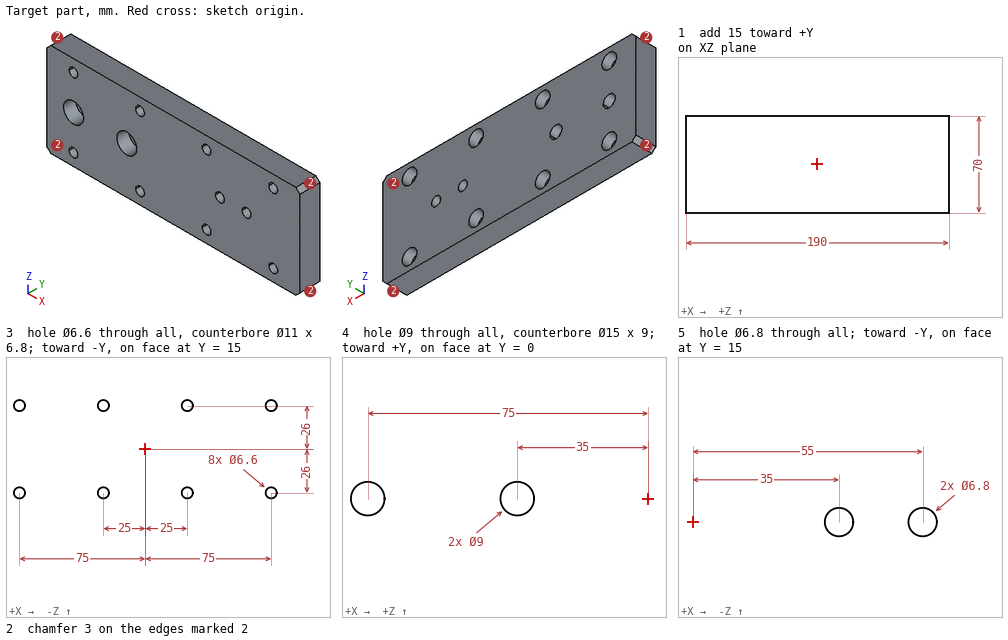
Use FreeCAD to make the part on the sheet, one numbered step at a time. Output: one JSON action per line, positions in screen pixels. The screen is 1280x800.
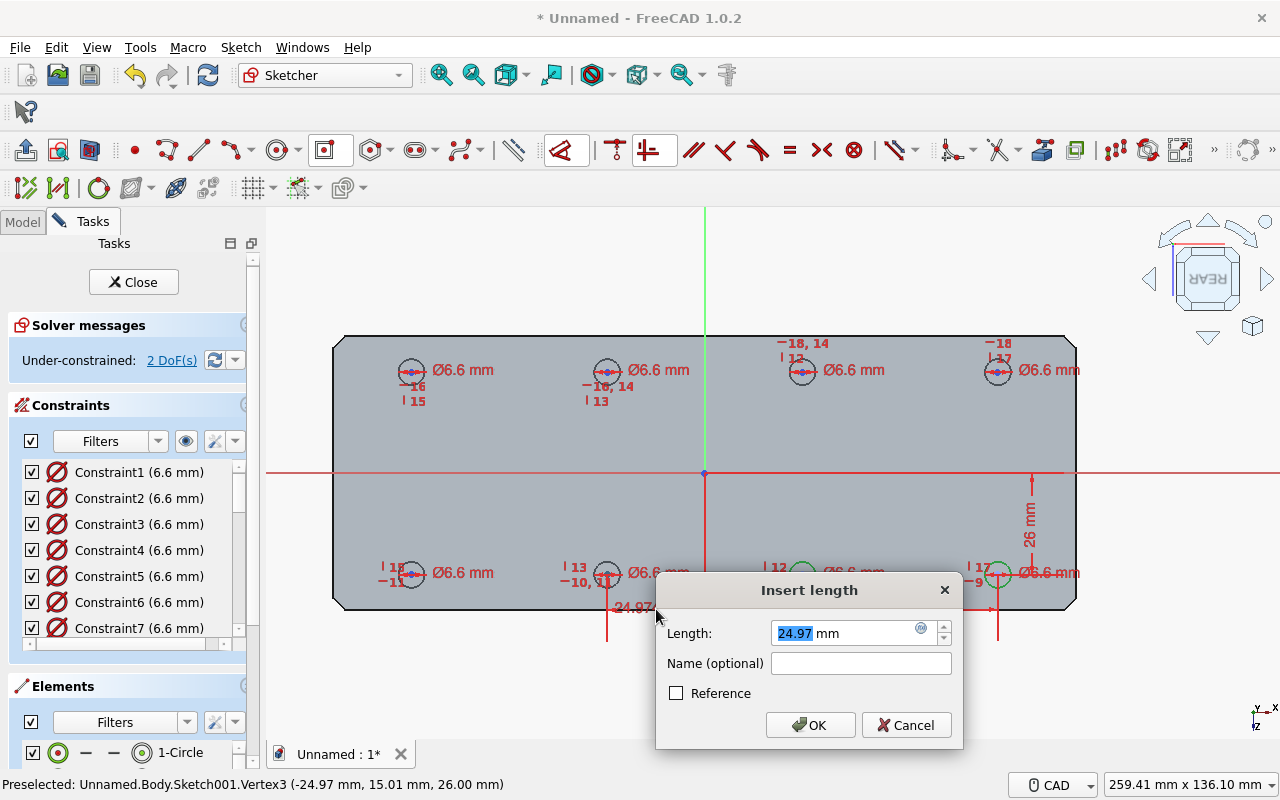
{"action": "type", "text": "25"}
{"action": "key", "text": "Return"}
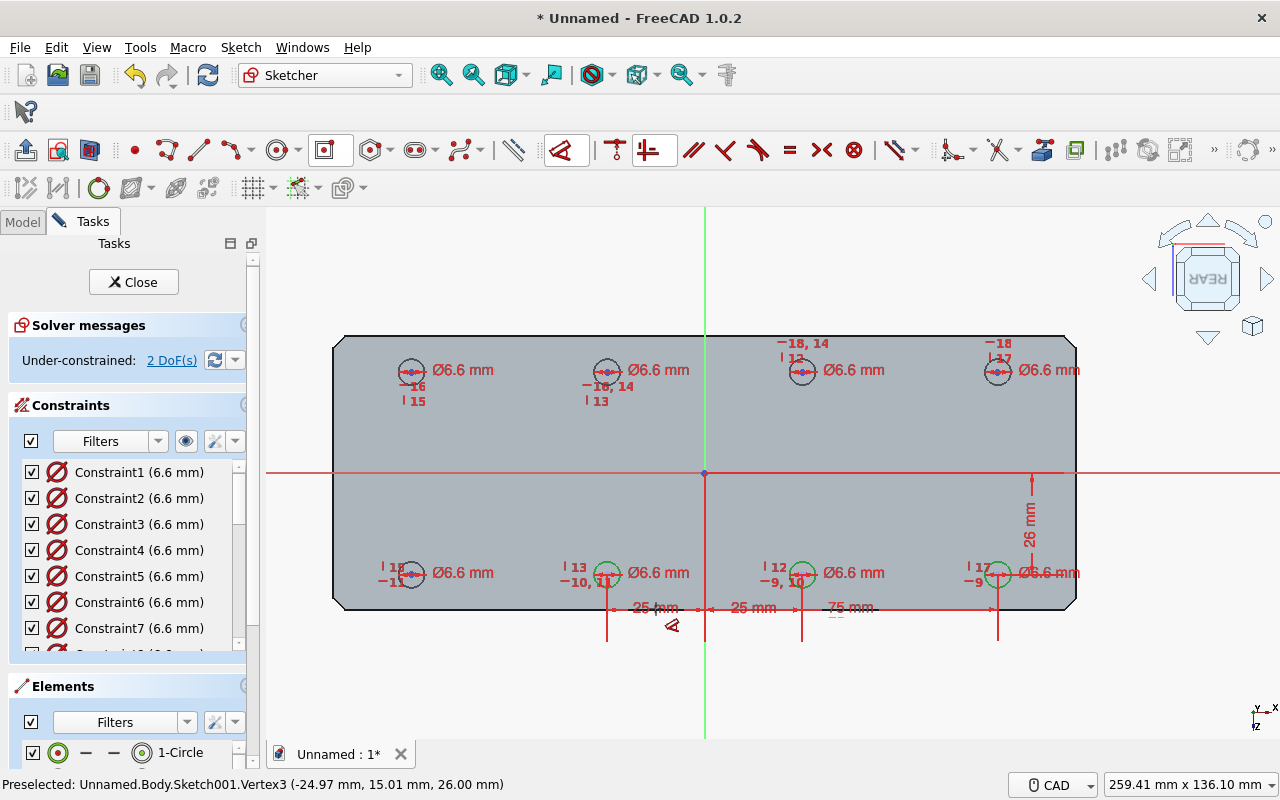
{"action": "left_click", "coordinate": [412, 575]}
{"action": "left_click", "coordinate": [558, 609]}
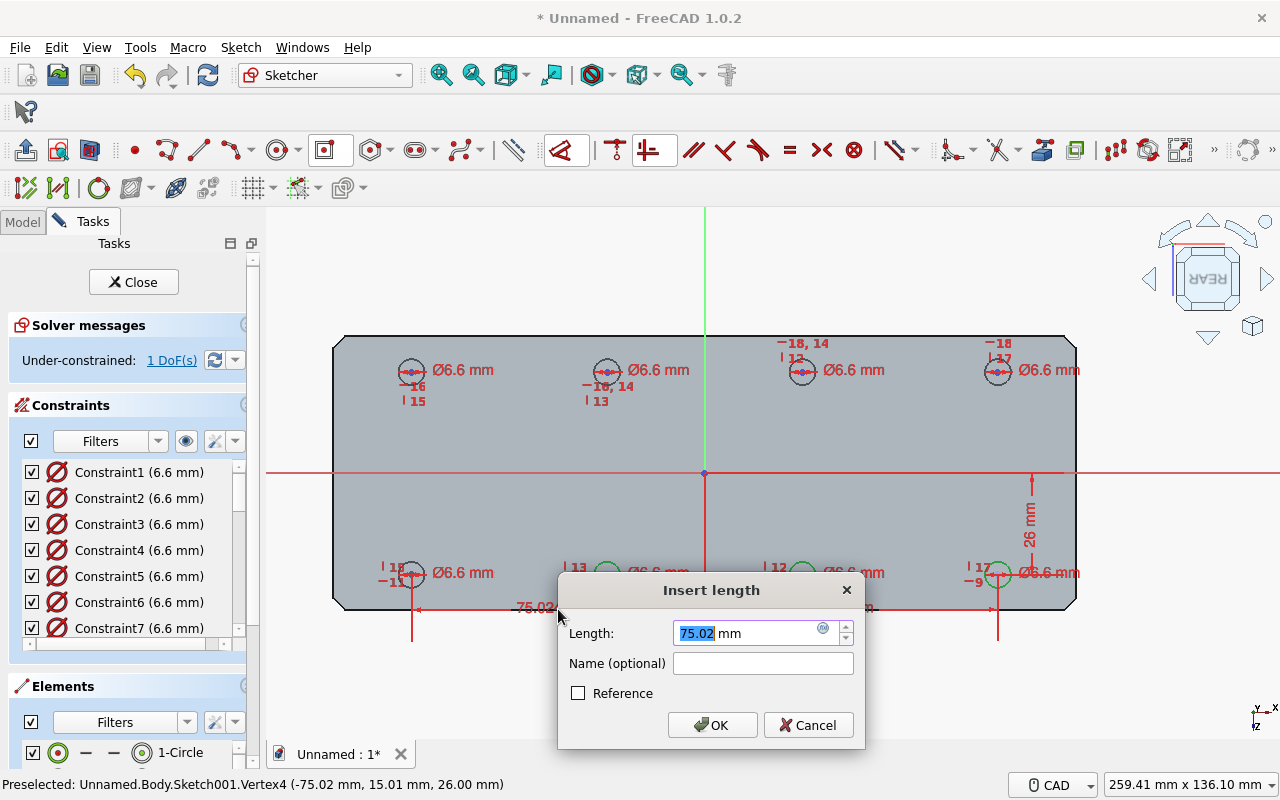
{"action": "type", "text": "75"}
{"action": "key", "text": "Return"}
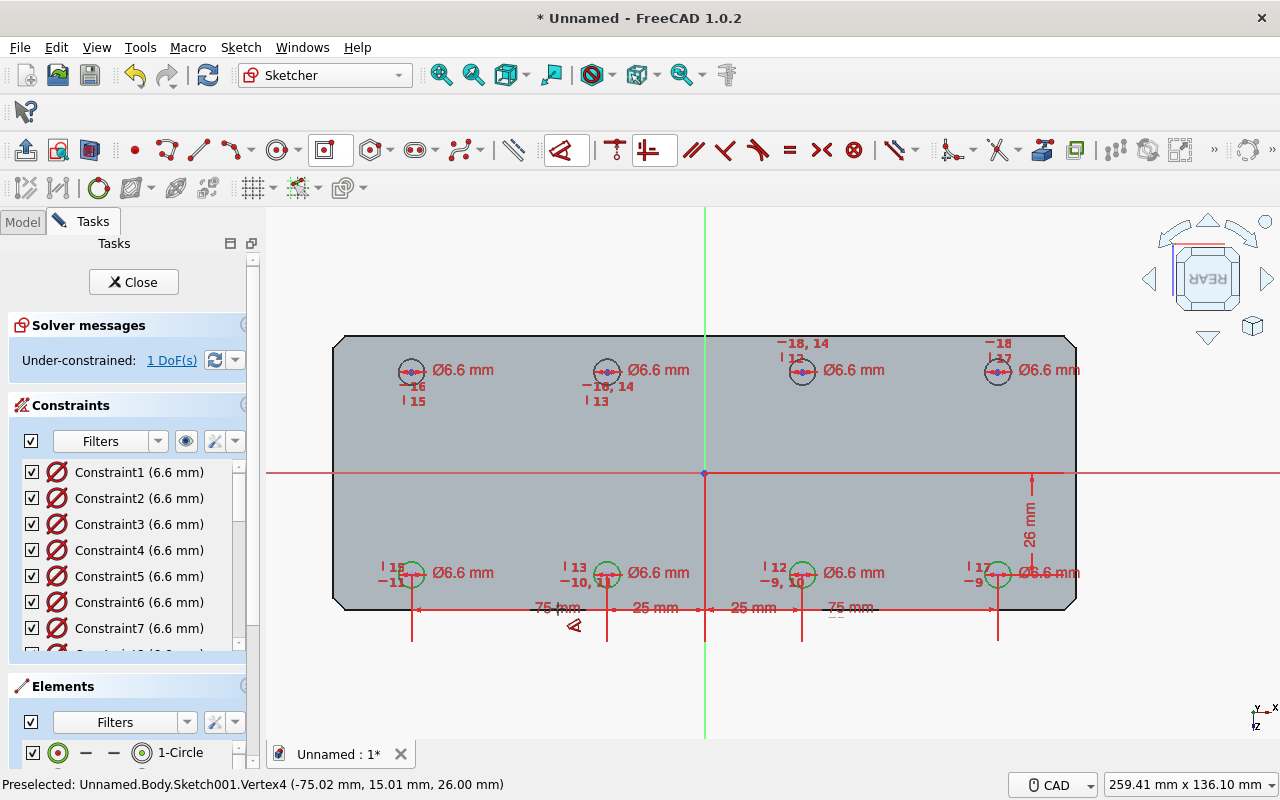
{"action": "left_click", "coordinate": [802, 372]}
{"action": "left_click", "coordinate": [836, 423]}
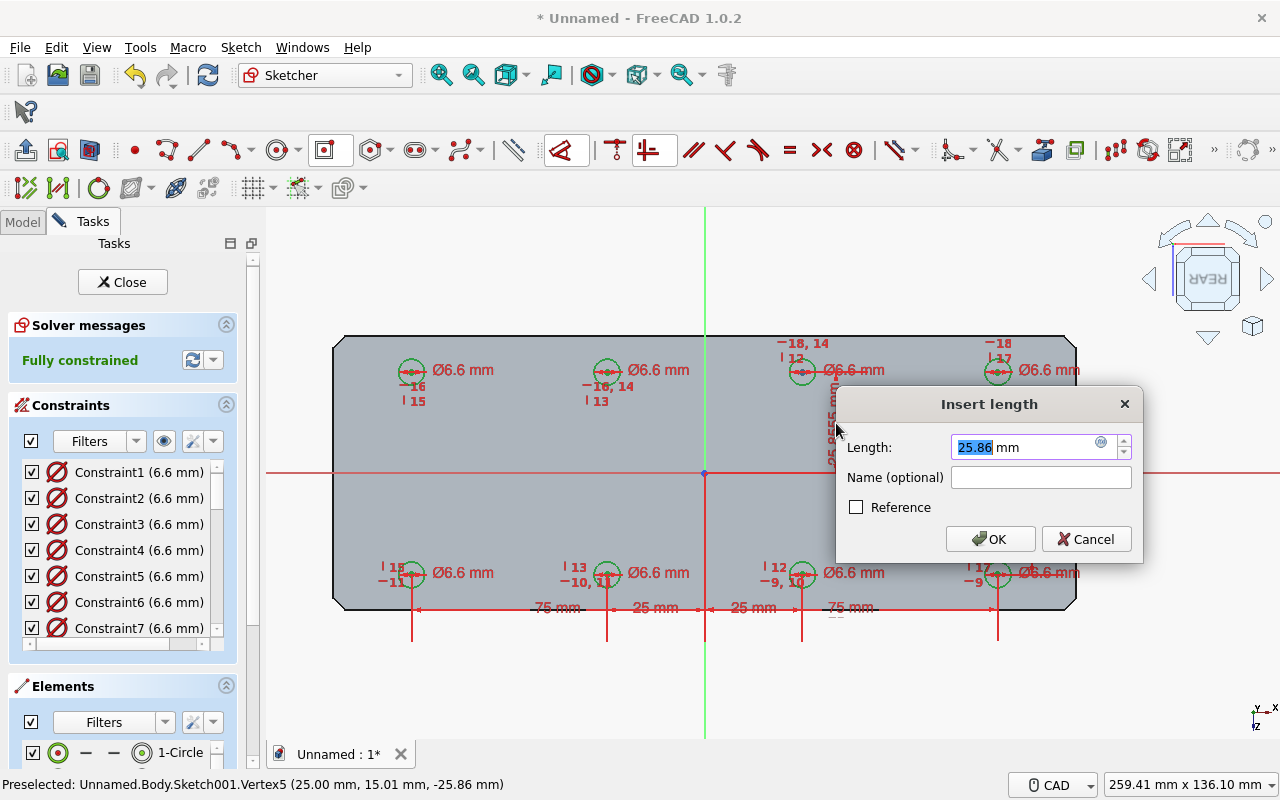
{"action": "type", "text": "26"}
{"action": "key", "text": "Return"}
{"action": "key", "text": "Escape"}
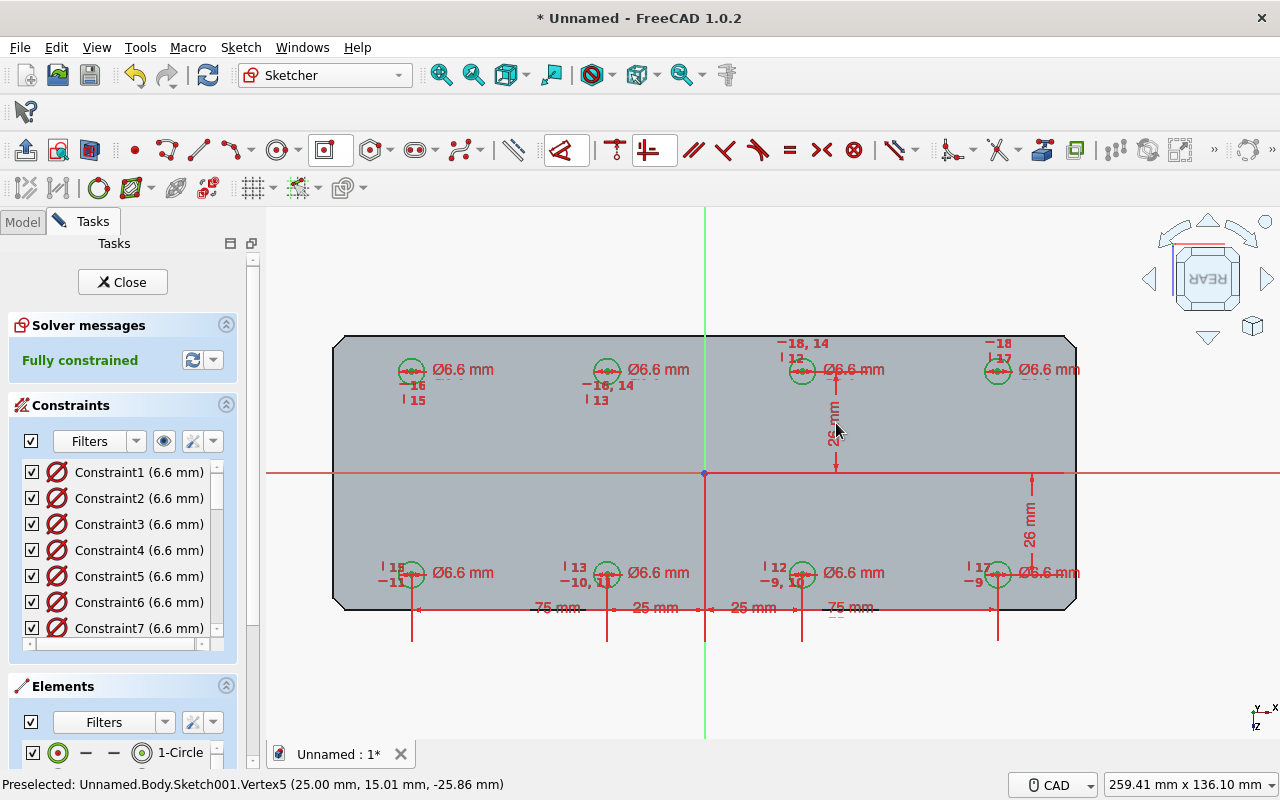
{"action": "left_click", "coordinate": [123, 282]}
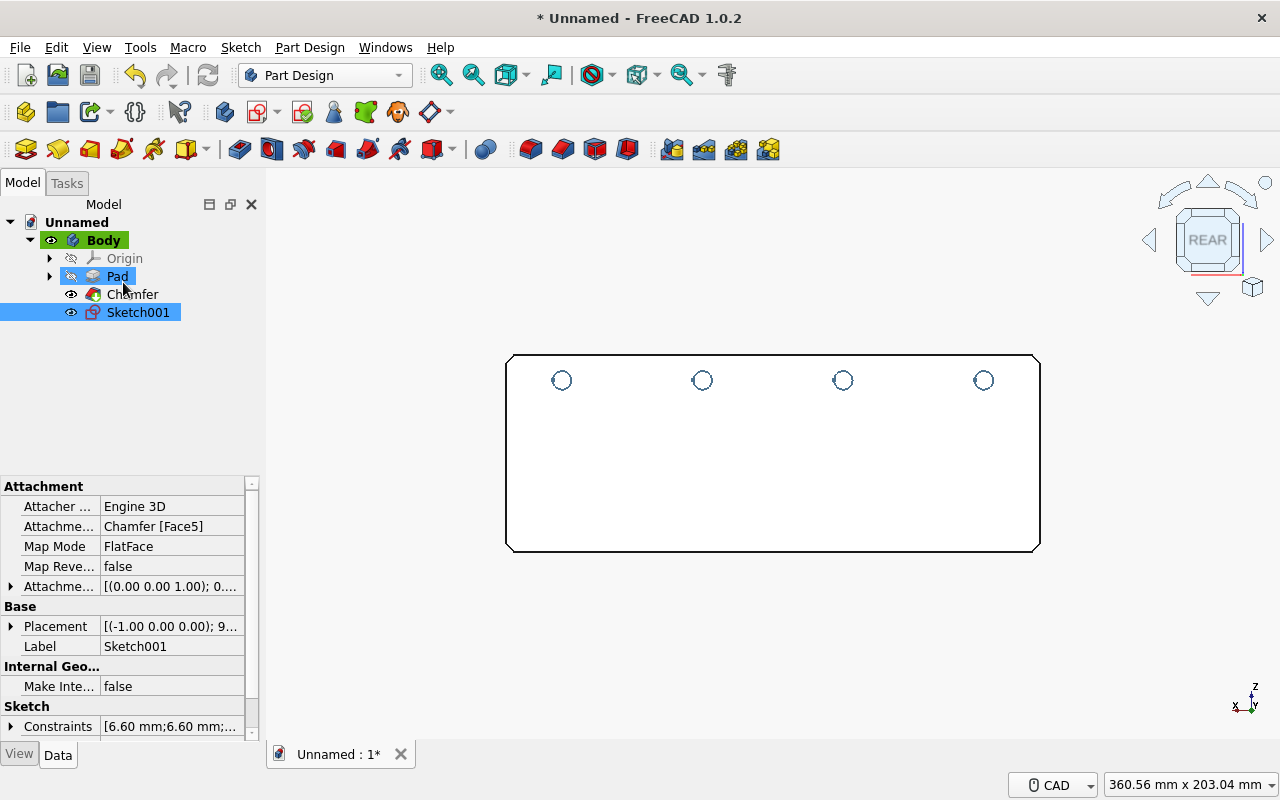
{"action": "left_click", "coordinate": [272, 150]}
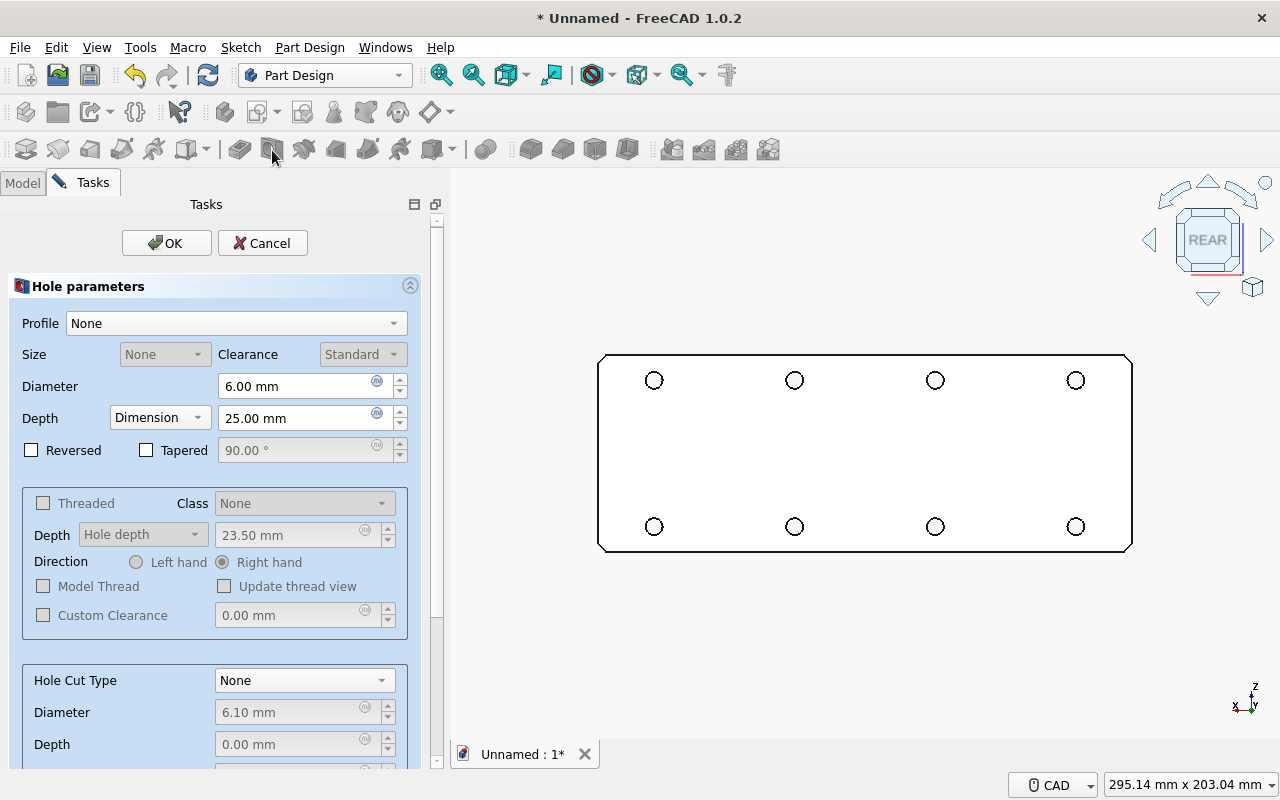
{"action": "triple_click", "coordinate": [305, 386]}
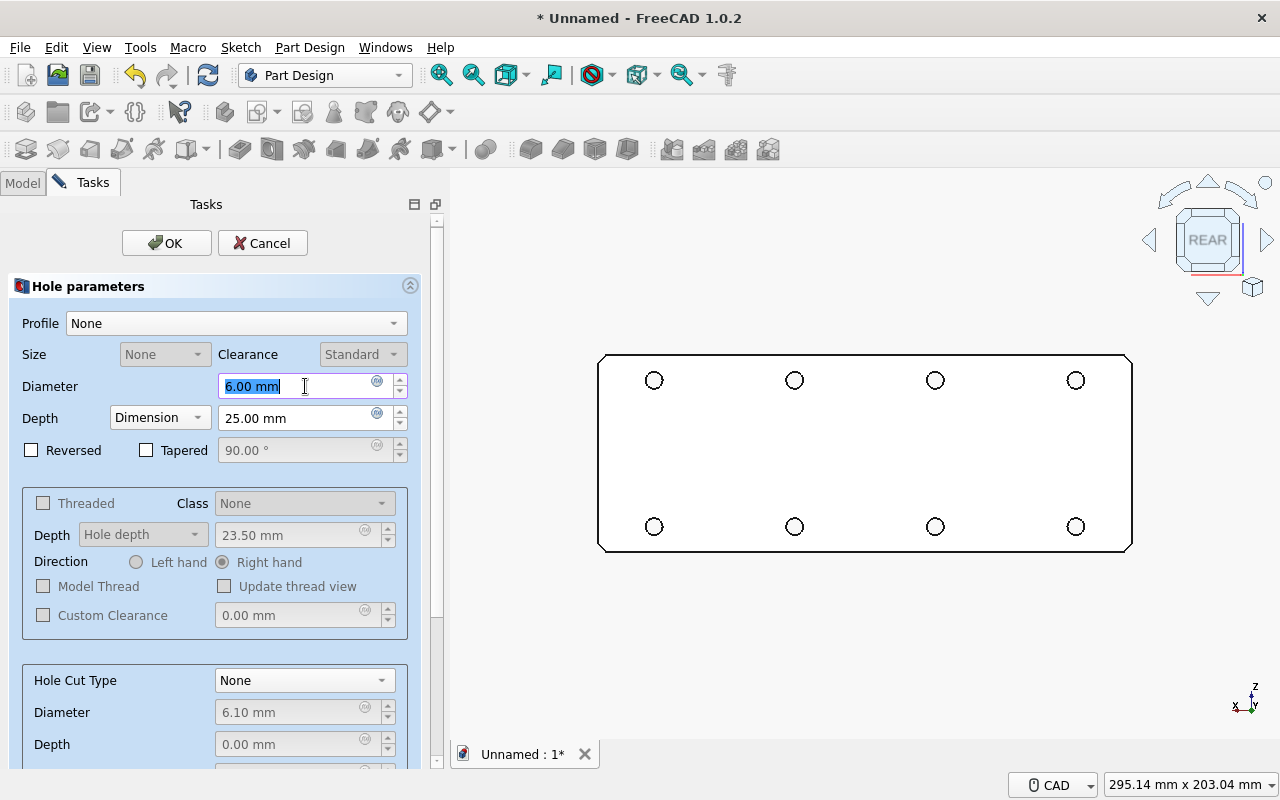
{"action": "type", "text": "6.6"}
{"action": "key", "text": "Tab"}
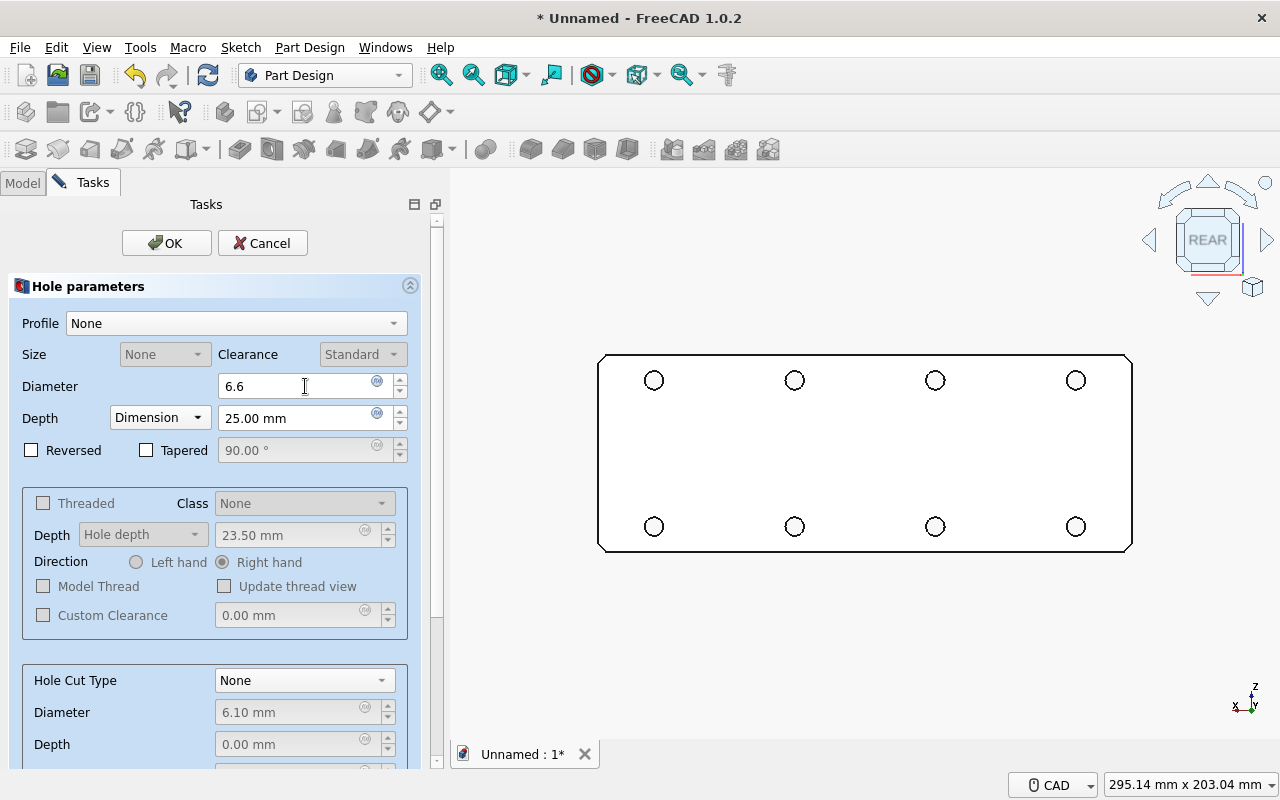
{"action": "left_click", "coordinate": [161, 418]}